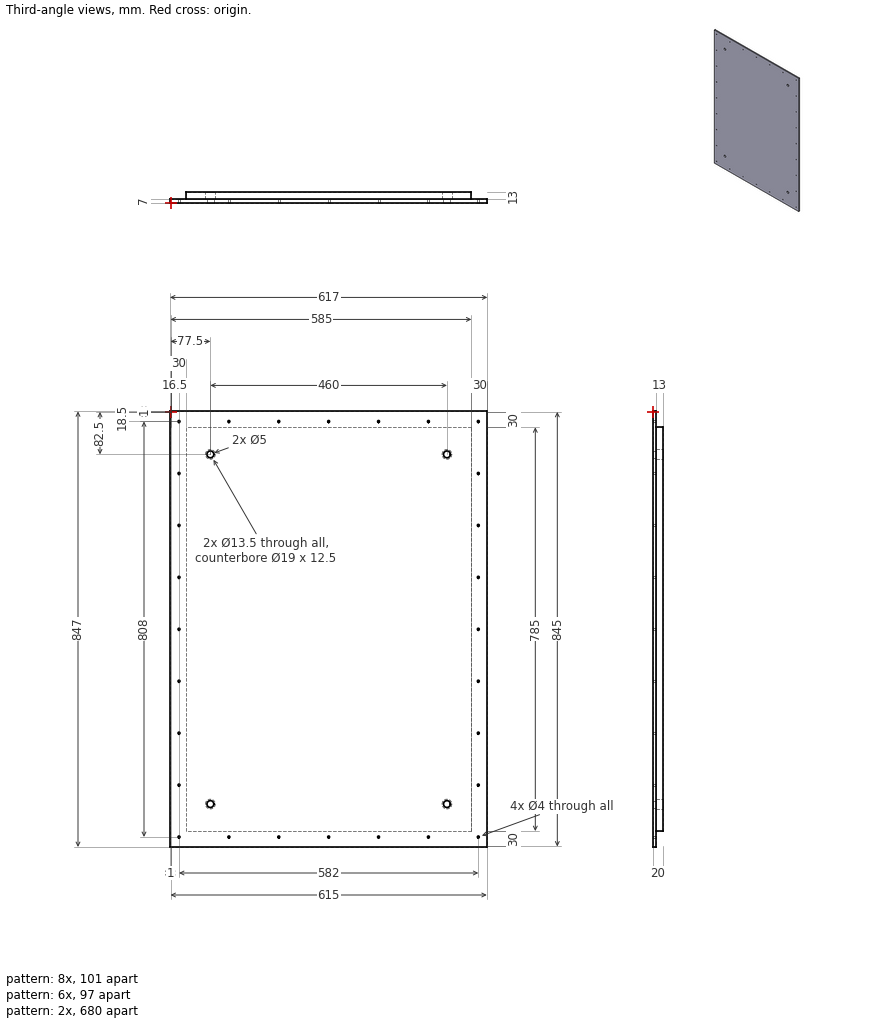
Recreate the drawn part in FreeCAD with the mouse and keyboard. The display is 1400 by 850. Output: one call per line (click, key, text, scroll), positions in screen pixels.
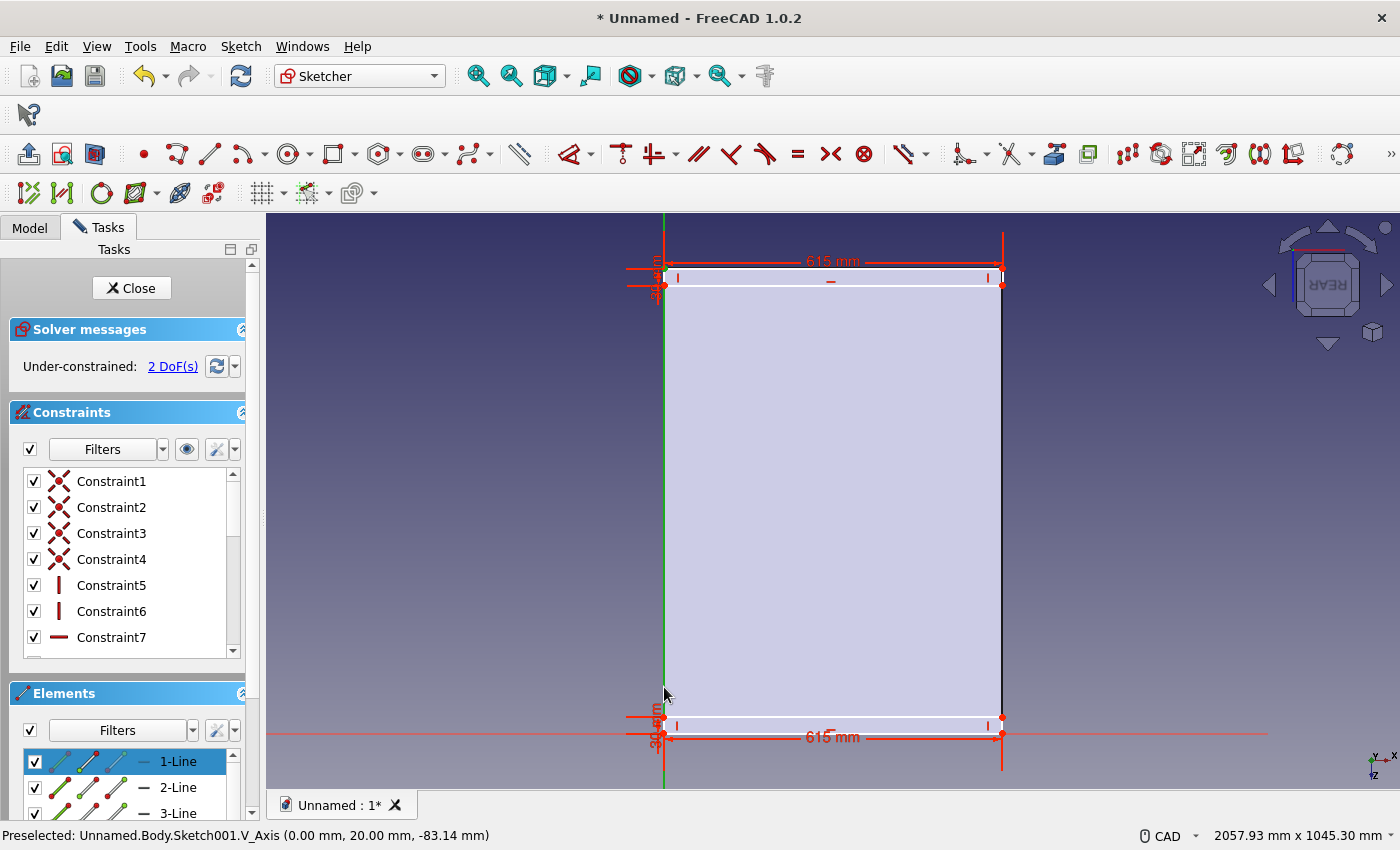
click(621, 154)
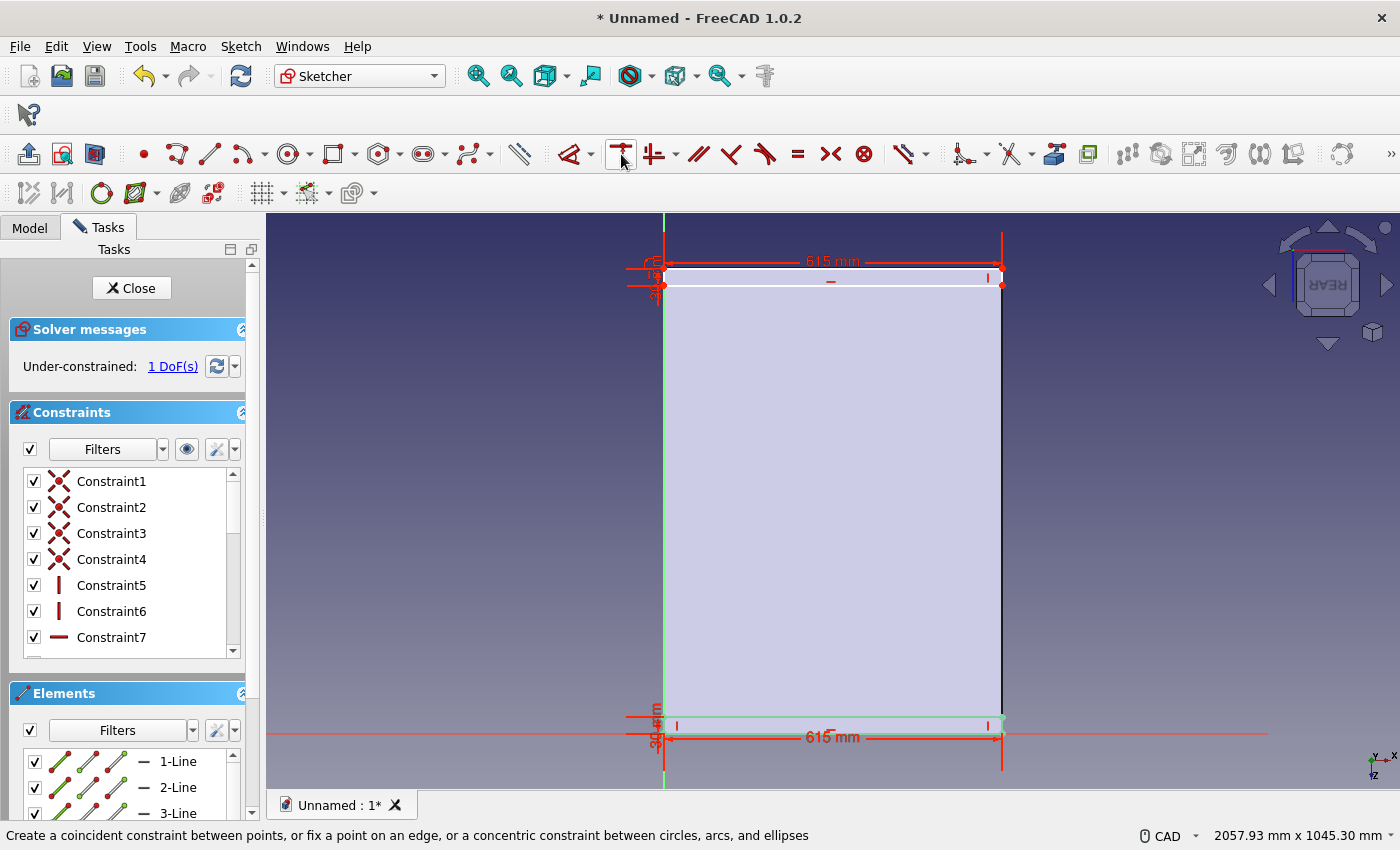
click(568, 154)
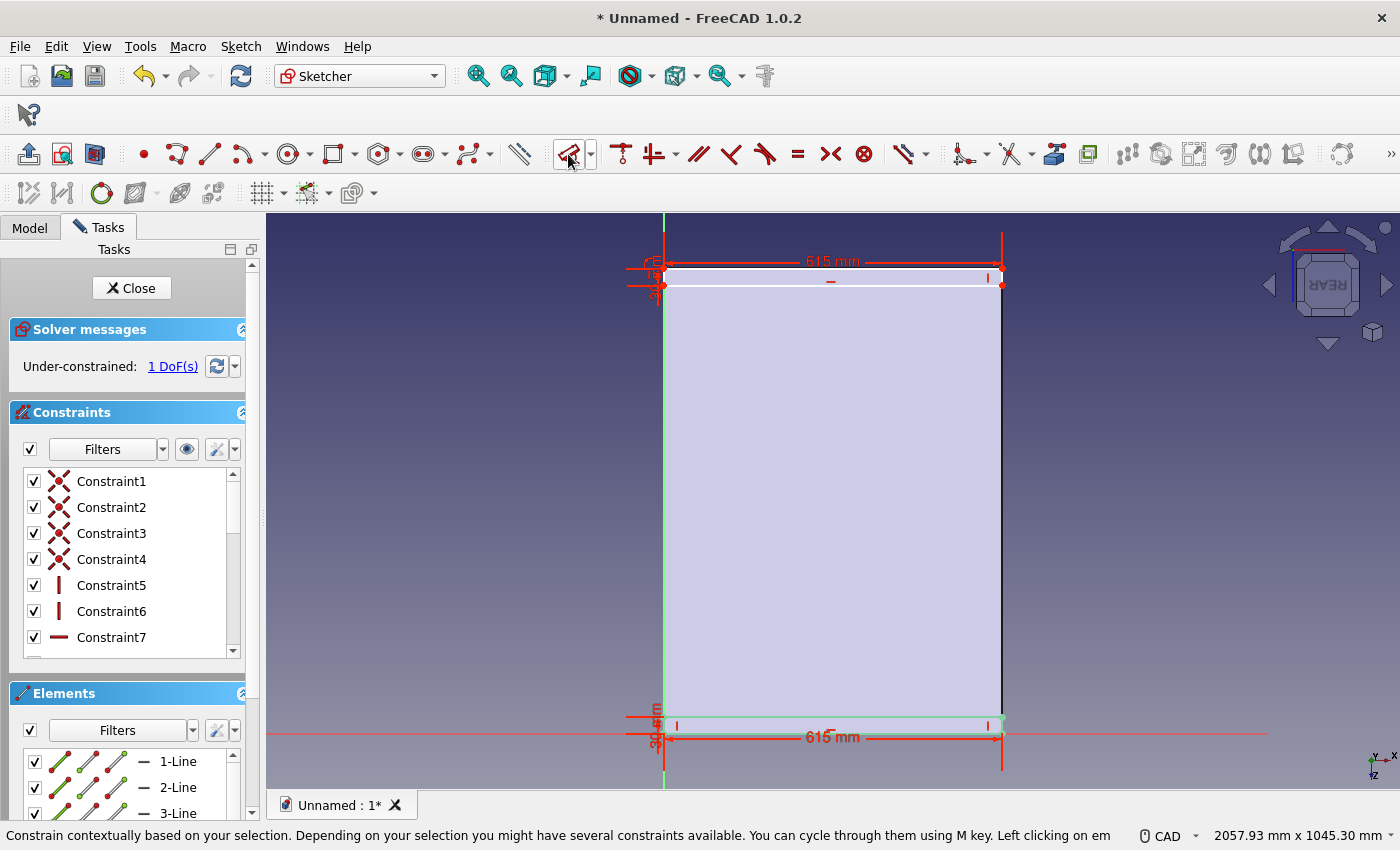
click(664, 269)
click(630, 501)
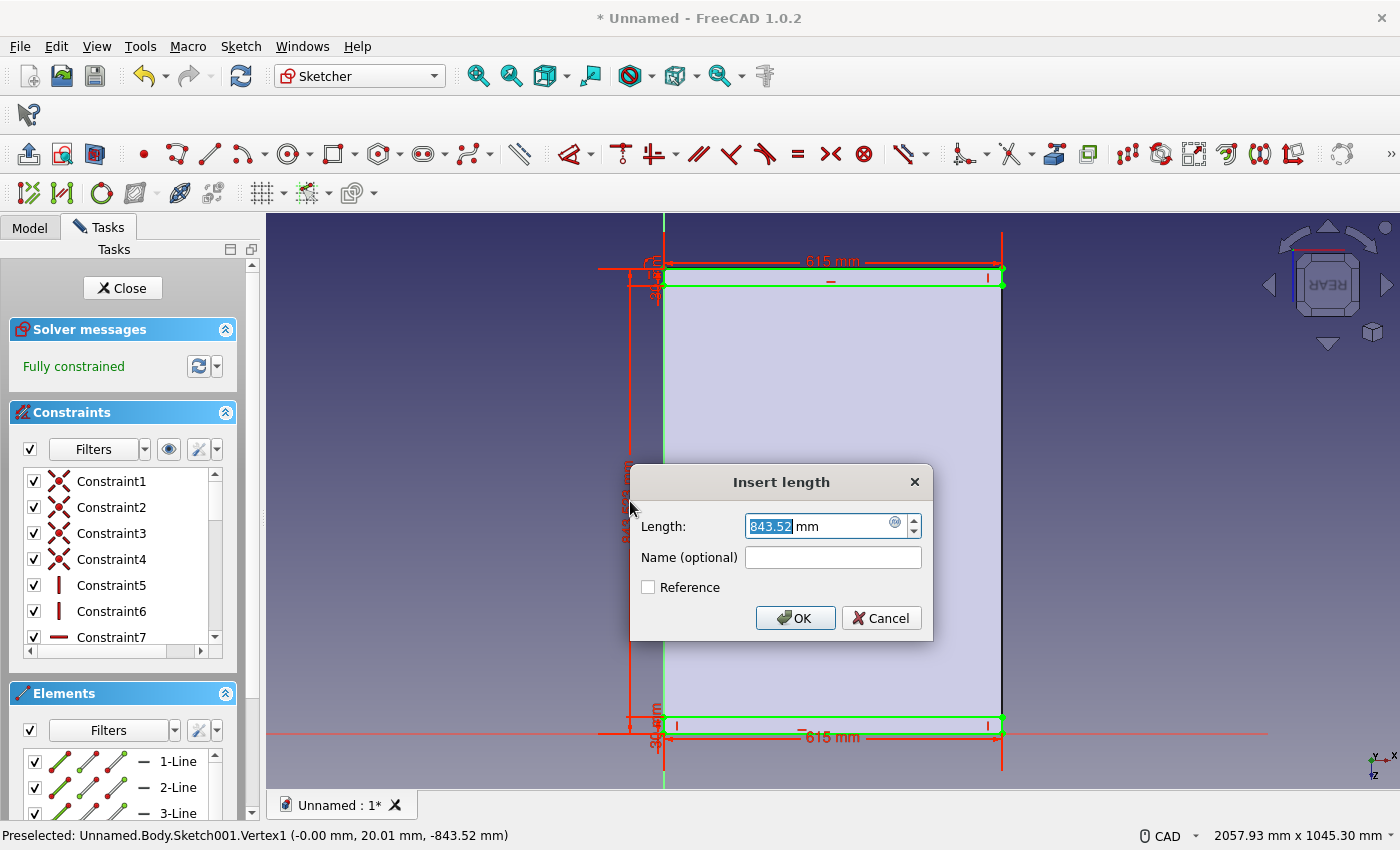
text(845)
key(Return)
key(Escape)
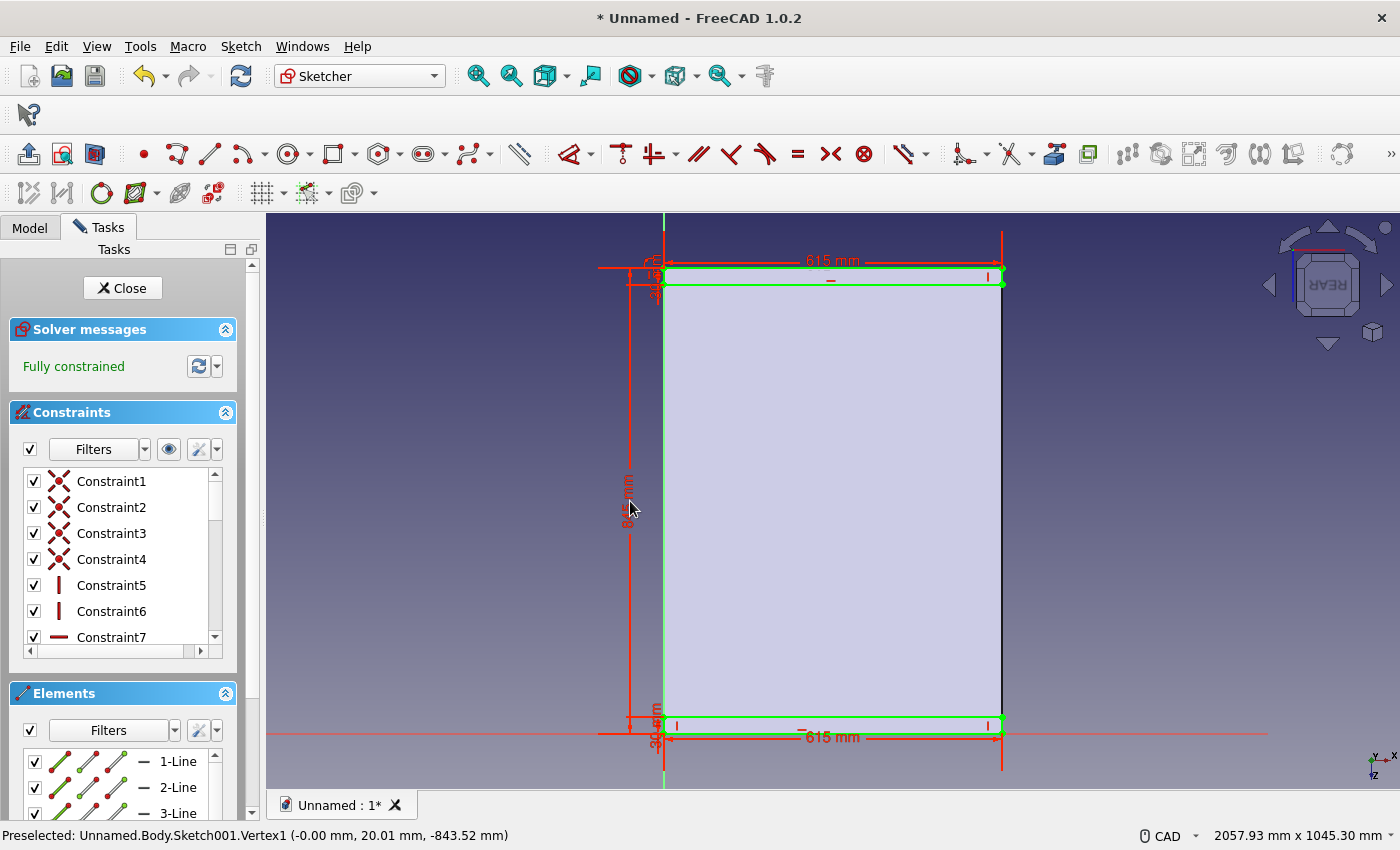
click(123, 288)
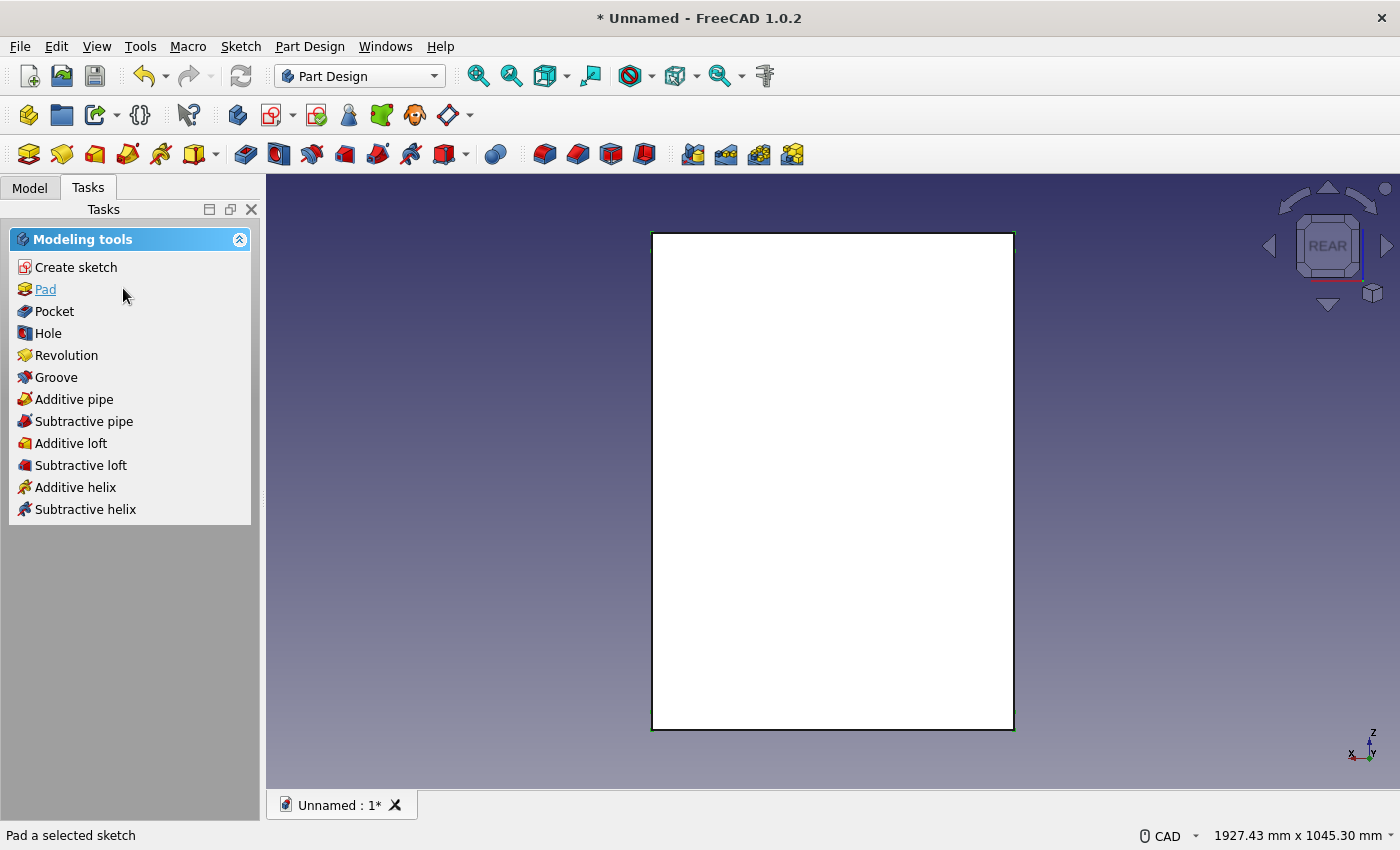
click(246, 154)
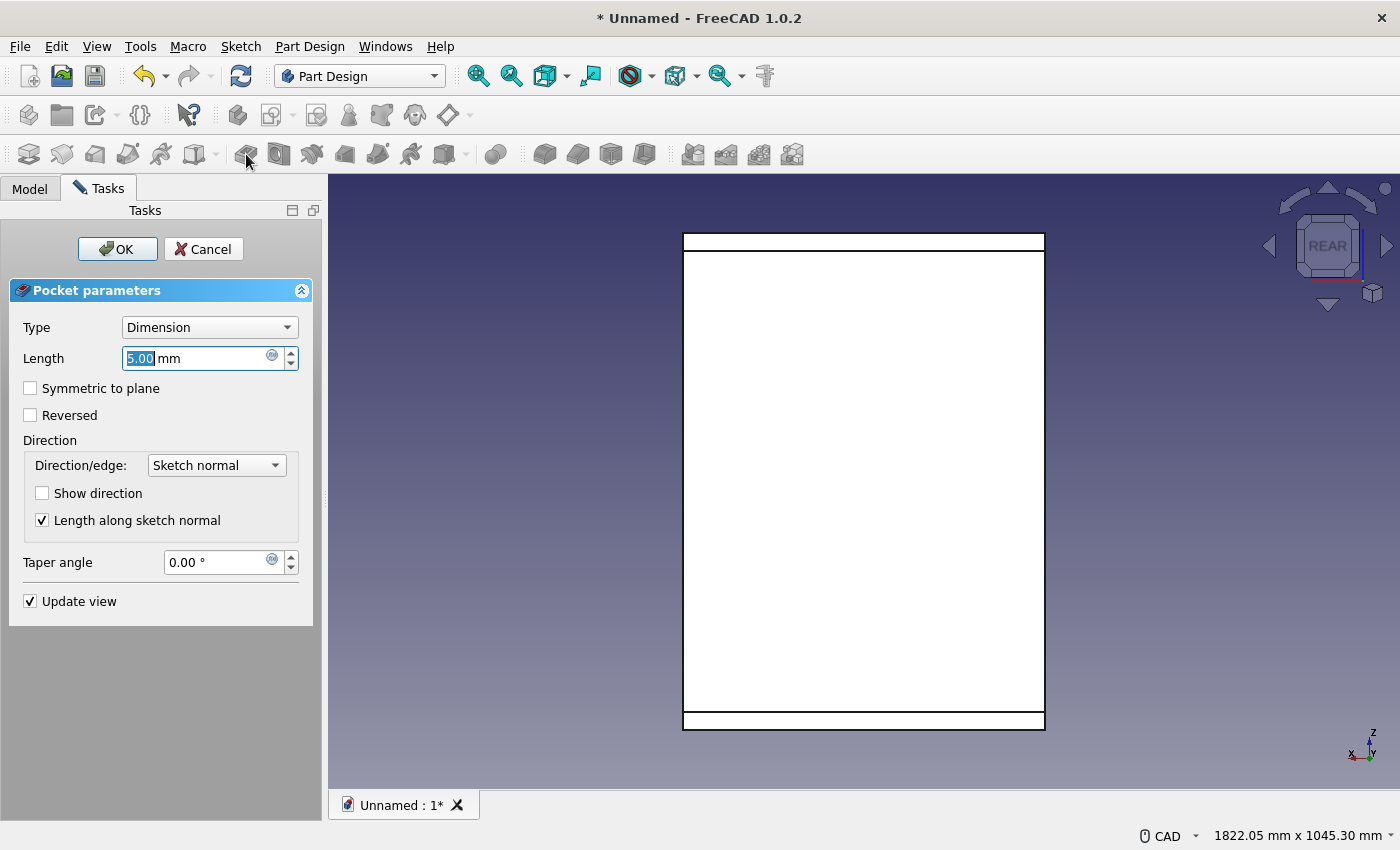
text(13)
key(Tab)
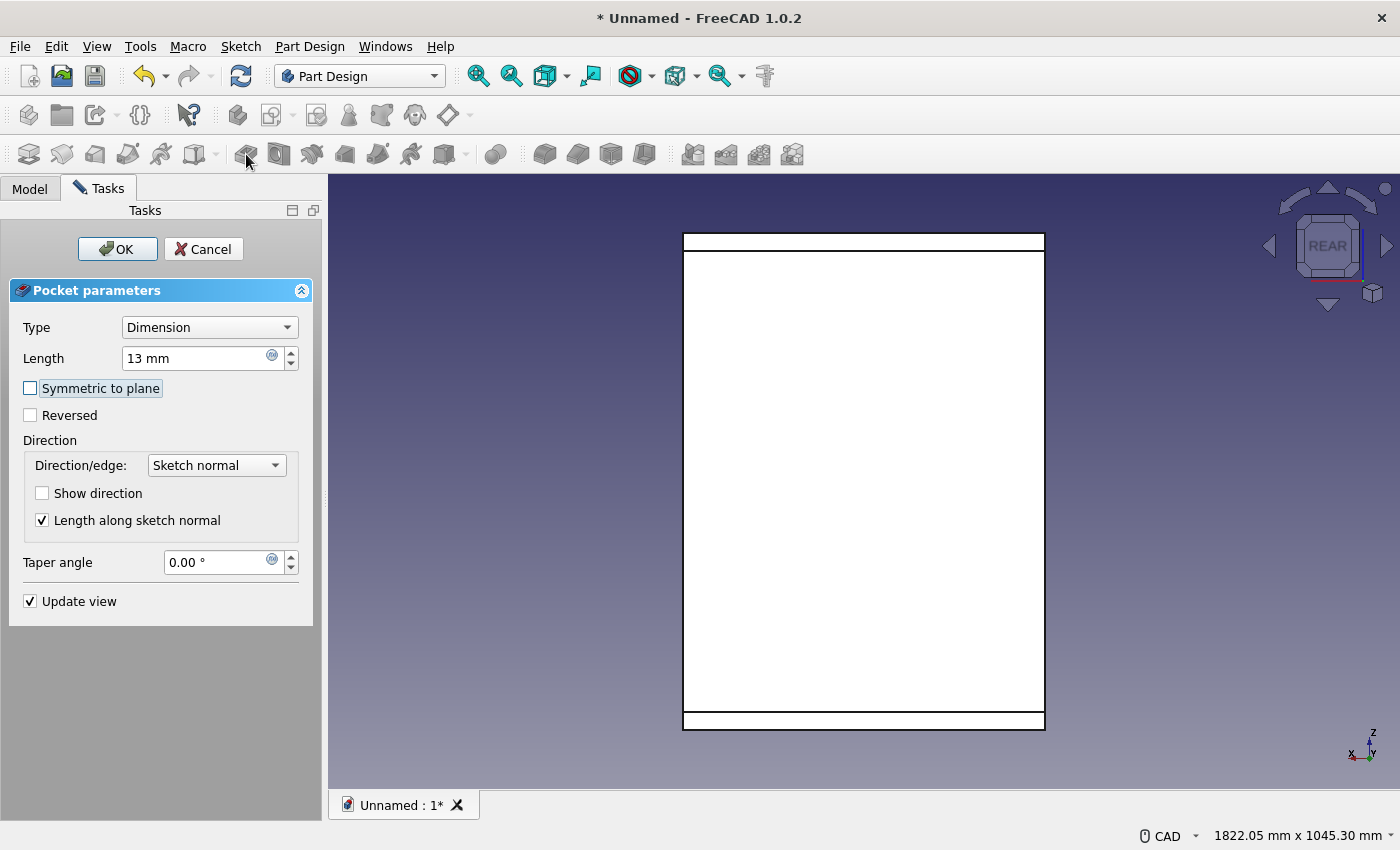
click(118, 249)